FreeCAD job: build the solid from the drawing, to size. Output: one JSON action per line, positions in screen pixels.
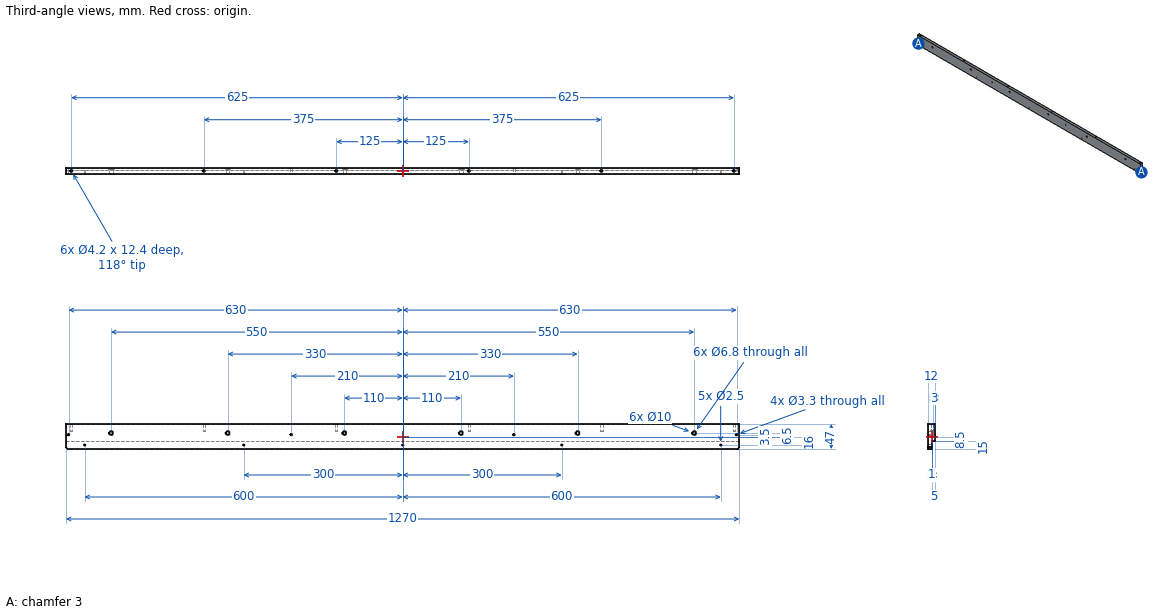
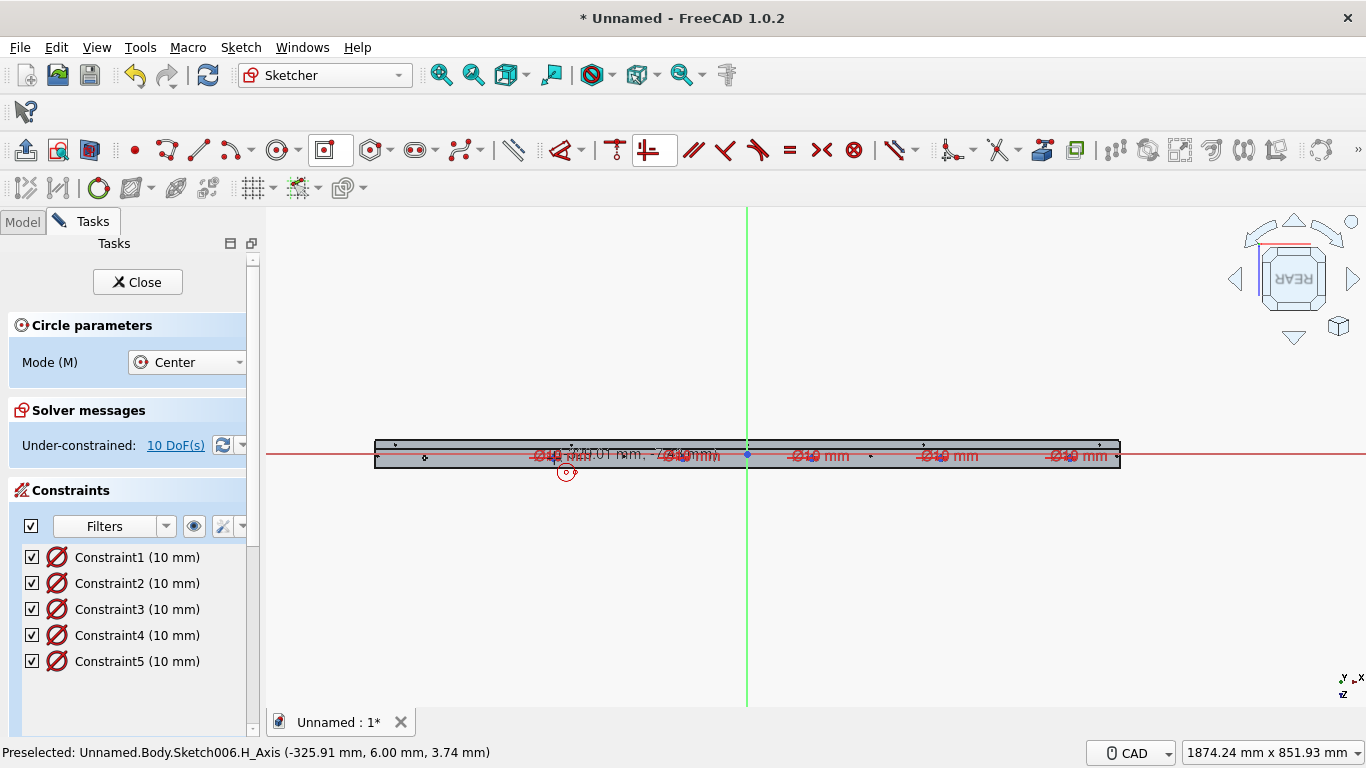
{"action": "scroll", "coordinate": [425, 458], "scroll_direction": "up", "scroll_amount": 11}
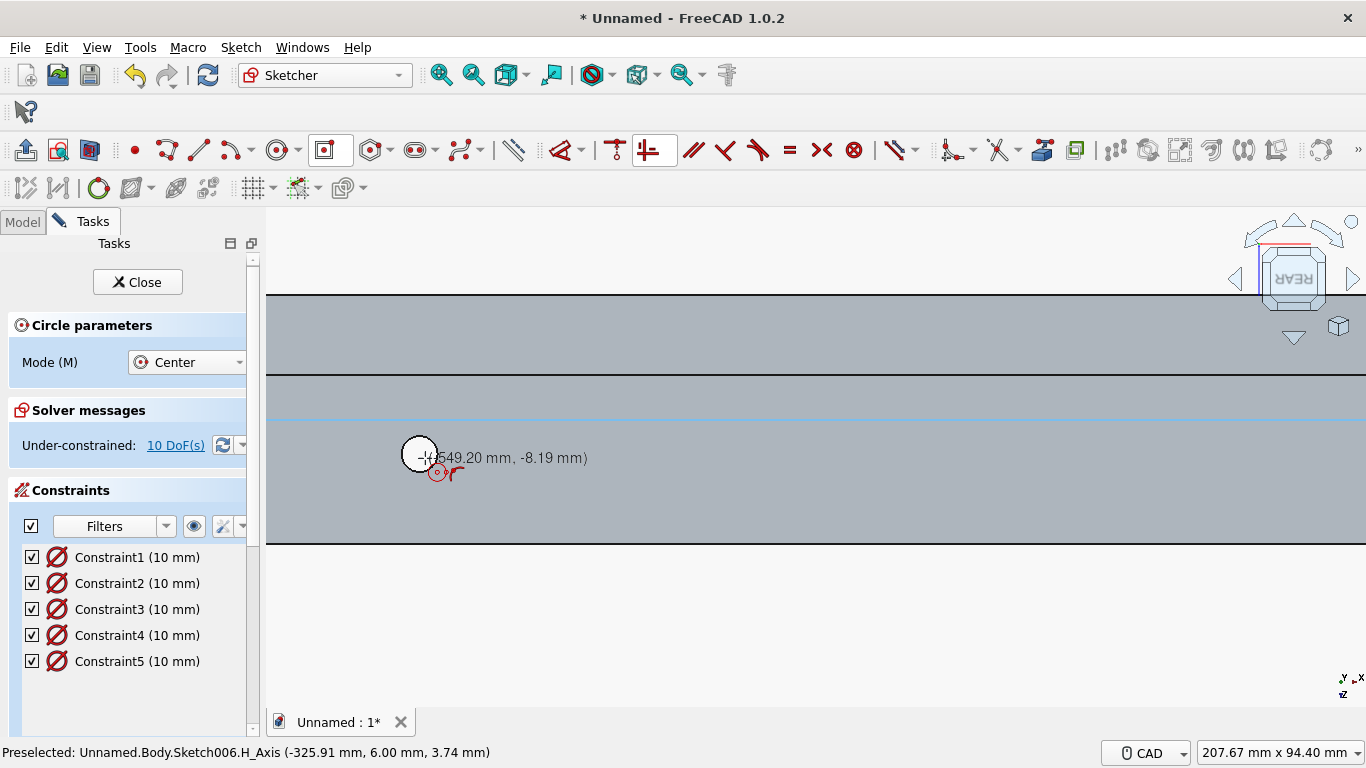
{"action": "left_click", "coordinate": [420, 454]}
{"action": "mouse_move", "coordinate": [438, 435]}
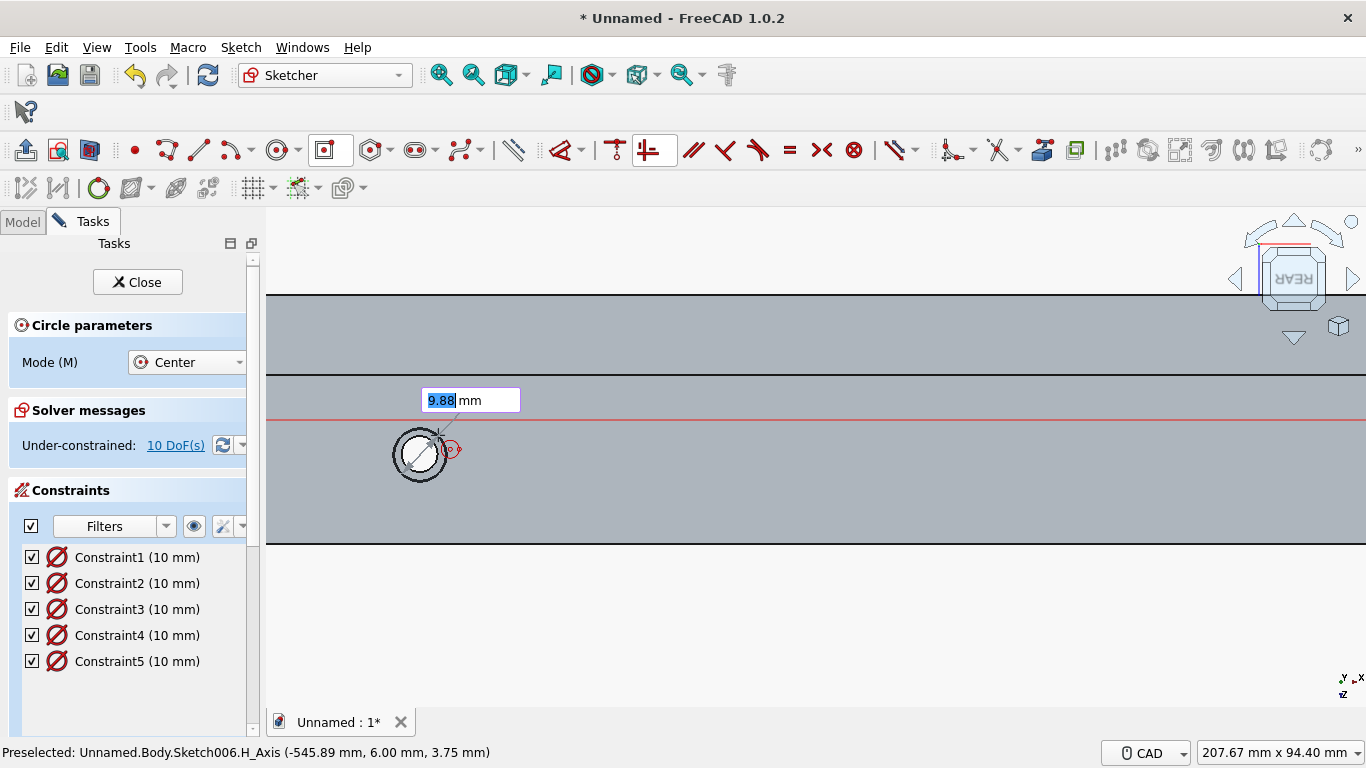
{"action": "type", "text": "10"}
{"action": "key", "text": "Return"}
{"action": "key", "text": "Escape"}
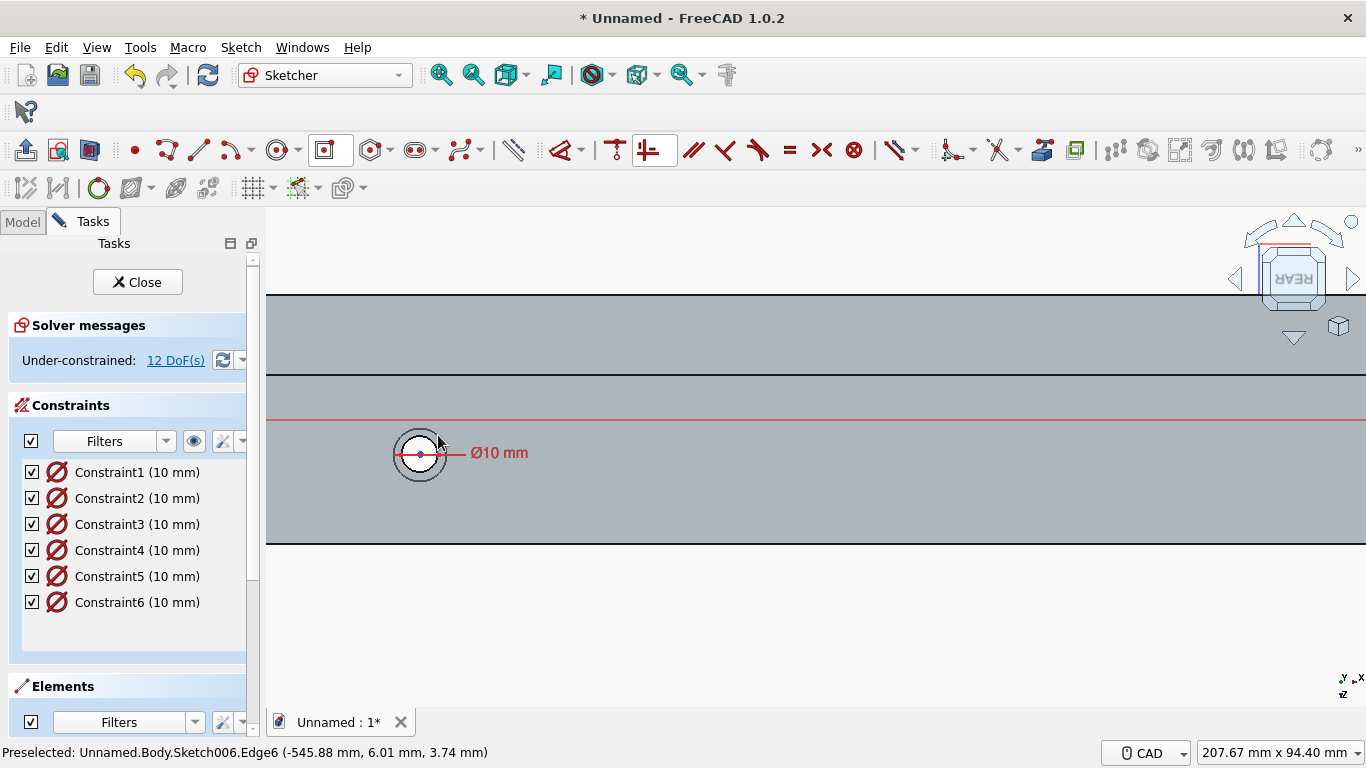
{"action": "scroll", "coordinate": [425, 458], "scroll_direction": "down", "scroll_amount": 11}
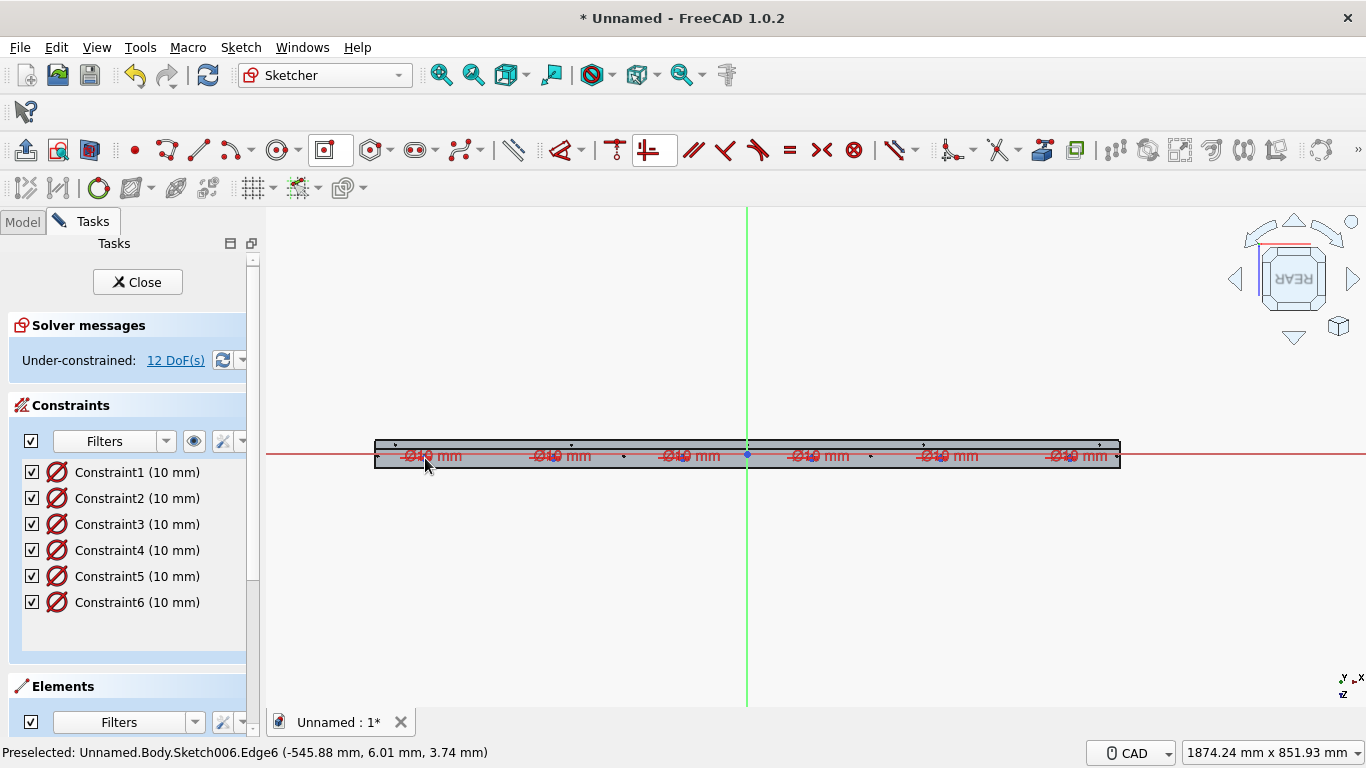
{"action": "left_click", "coordinate": [1070, 458]}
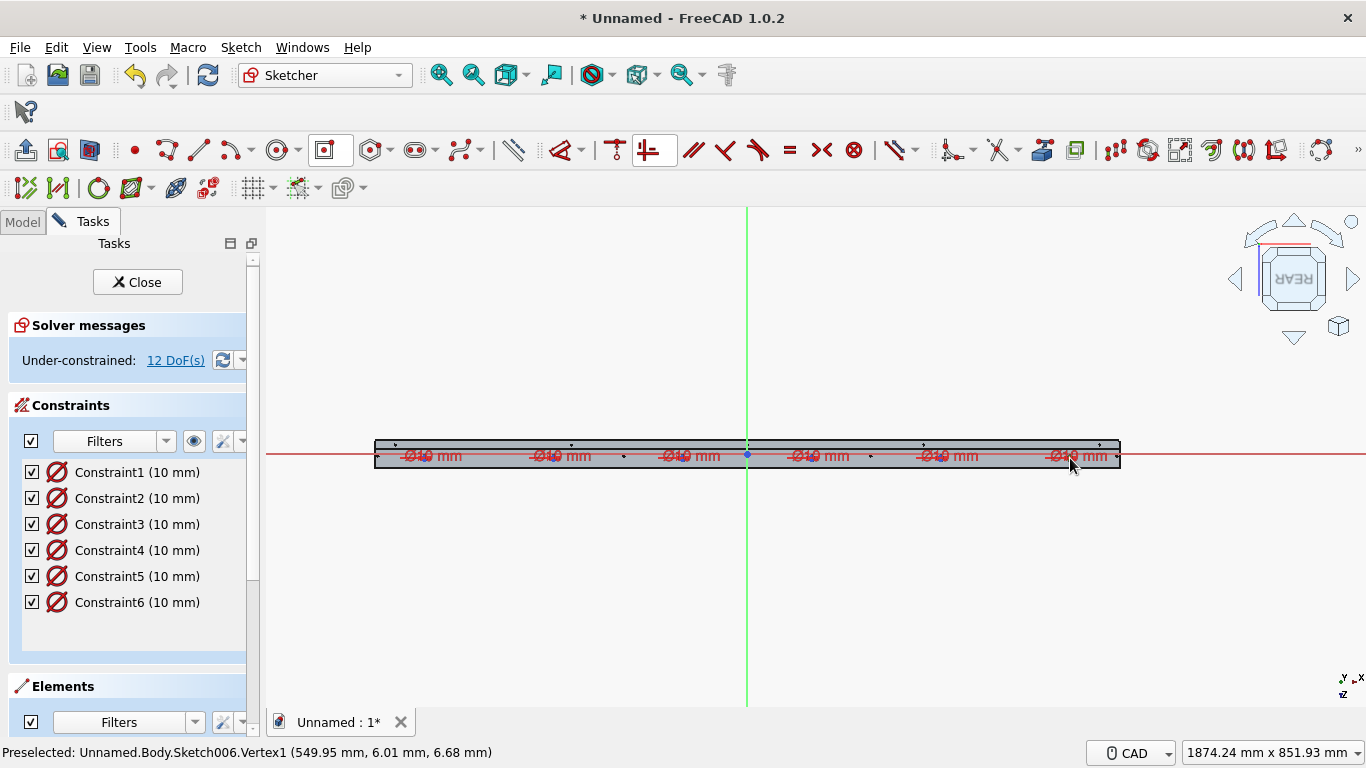
{"action": "left_click", "coordinate": [941, 458]}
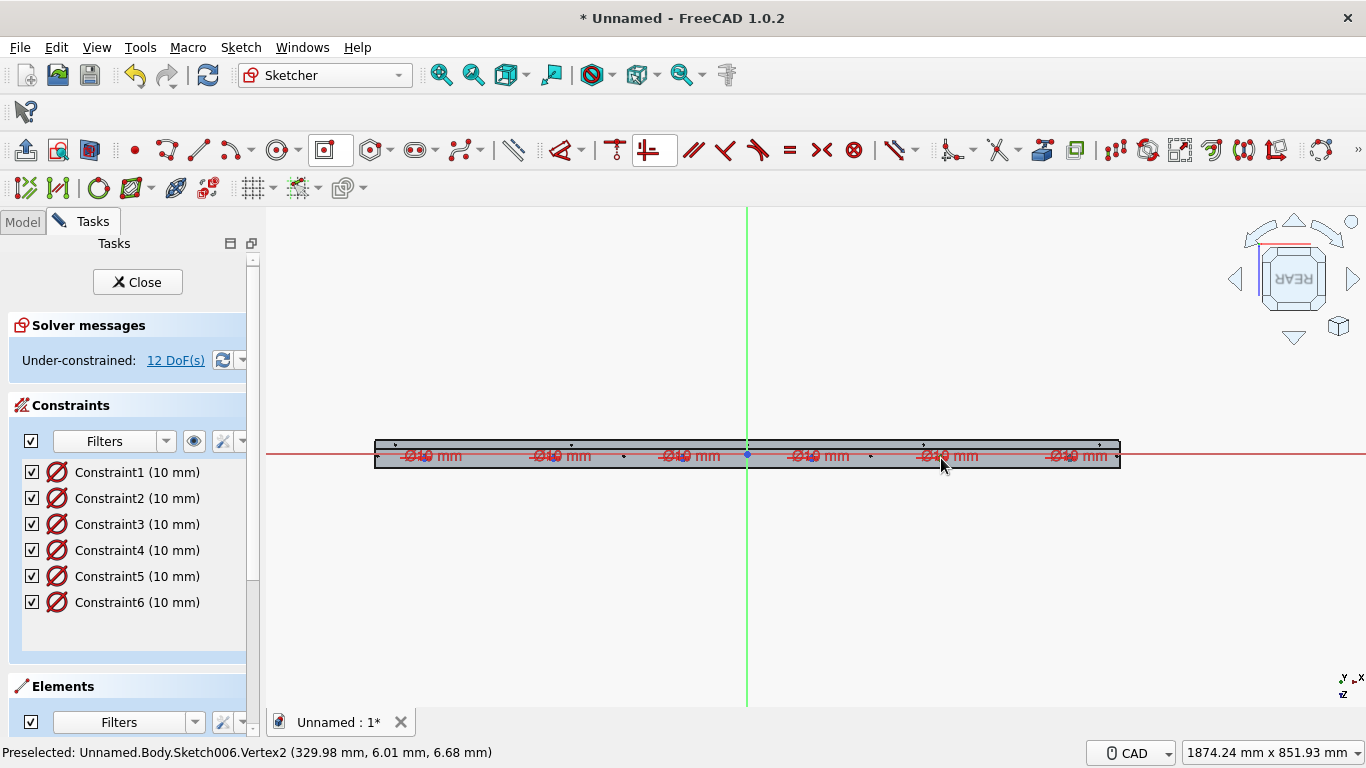
{"action": "left_click", "coordinate": [672, 150]}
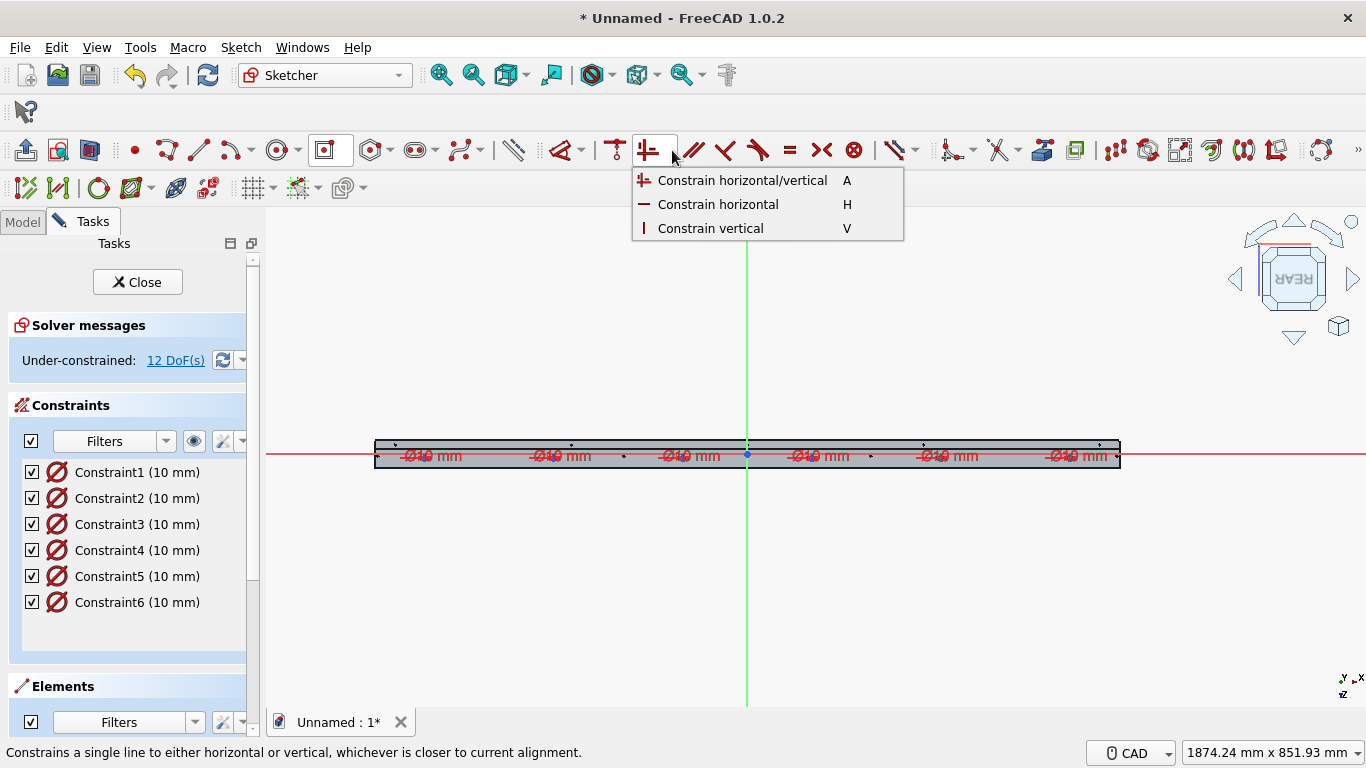
{"action": "left_click", "coordinate": [768, 204]}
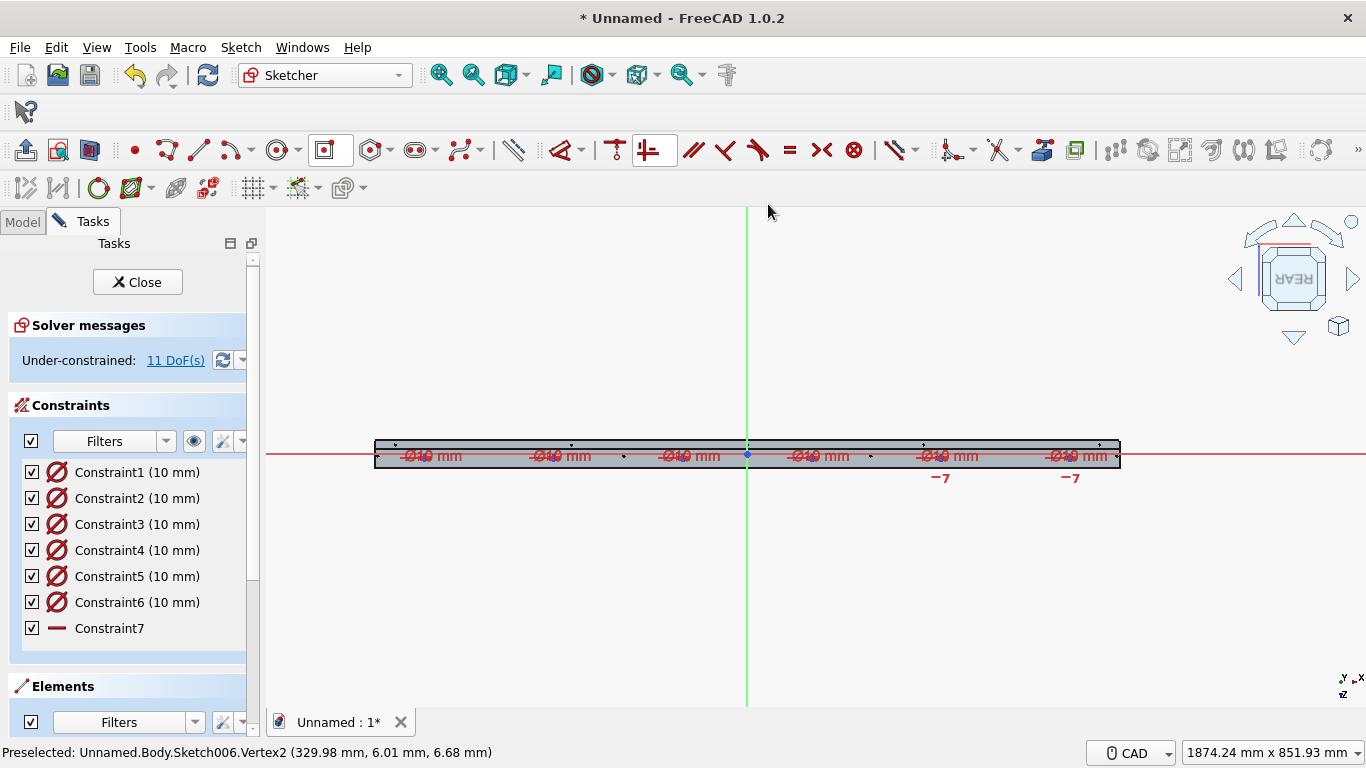
{"action": "left_click", "coordinate": [941, 458]}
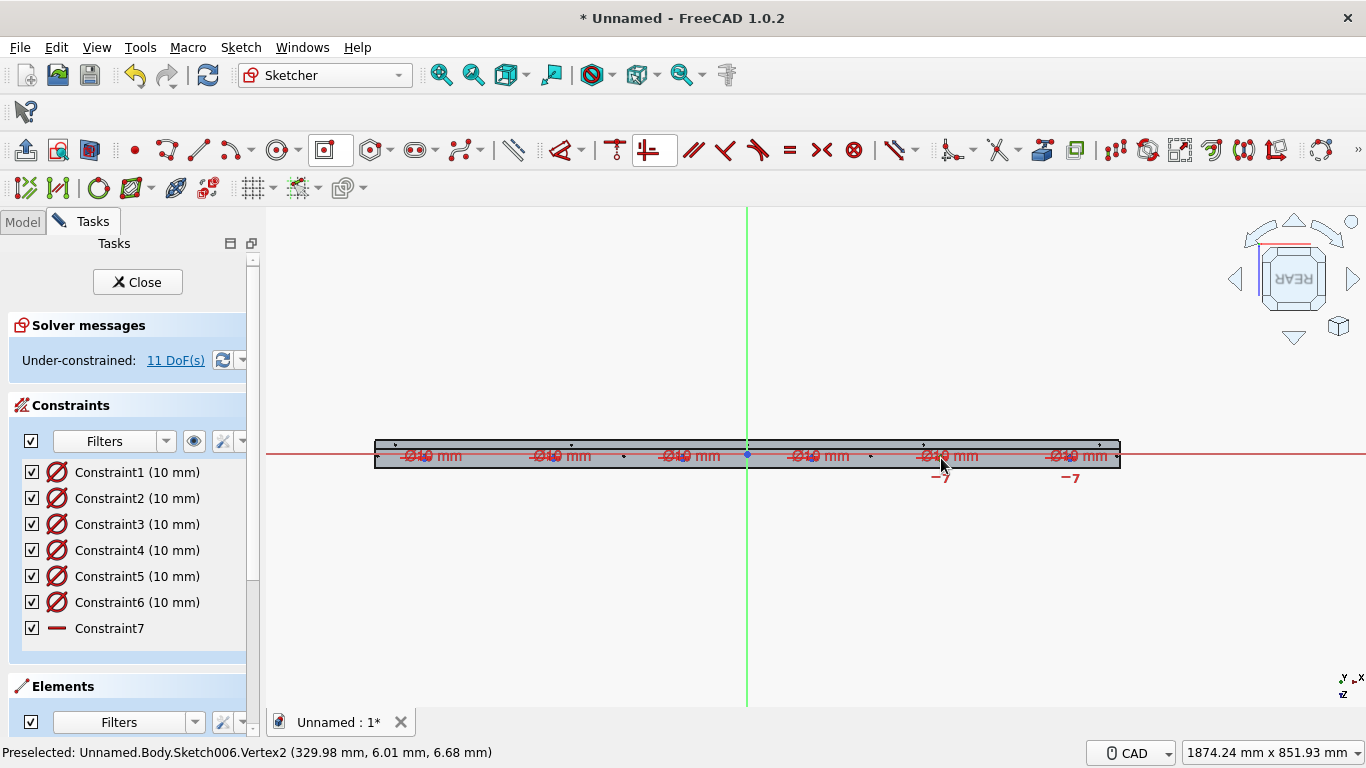
{"action": "left_click", "coordinate": [812, 458]}